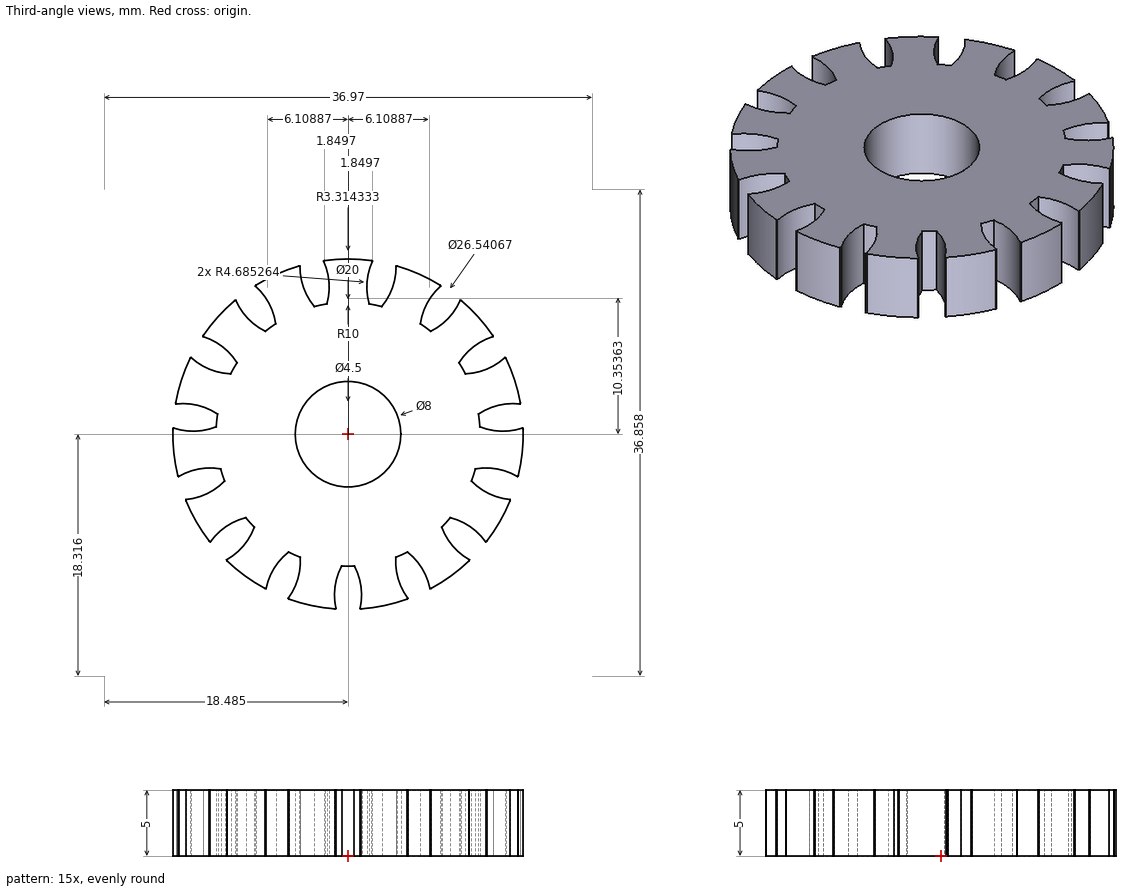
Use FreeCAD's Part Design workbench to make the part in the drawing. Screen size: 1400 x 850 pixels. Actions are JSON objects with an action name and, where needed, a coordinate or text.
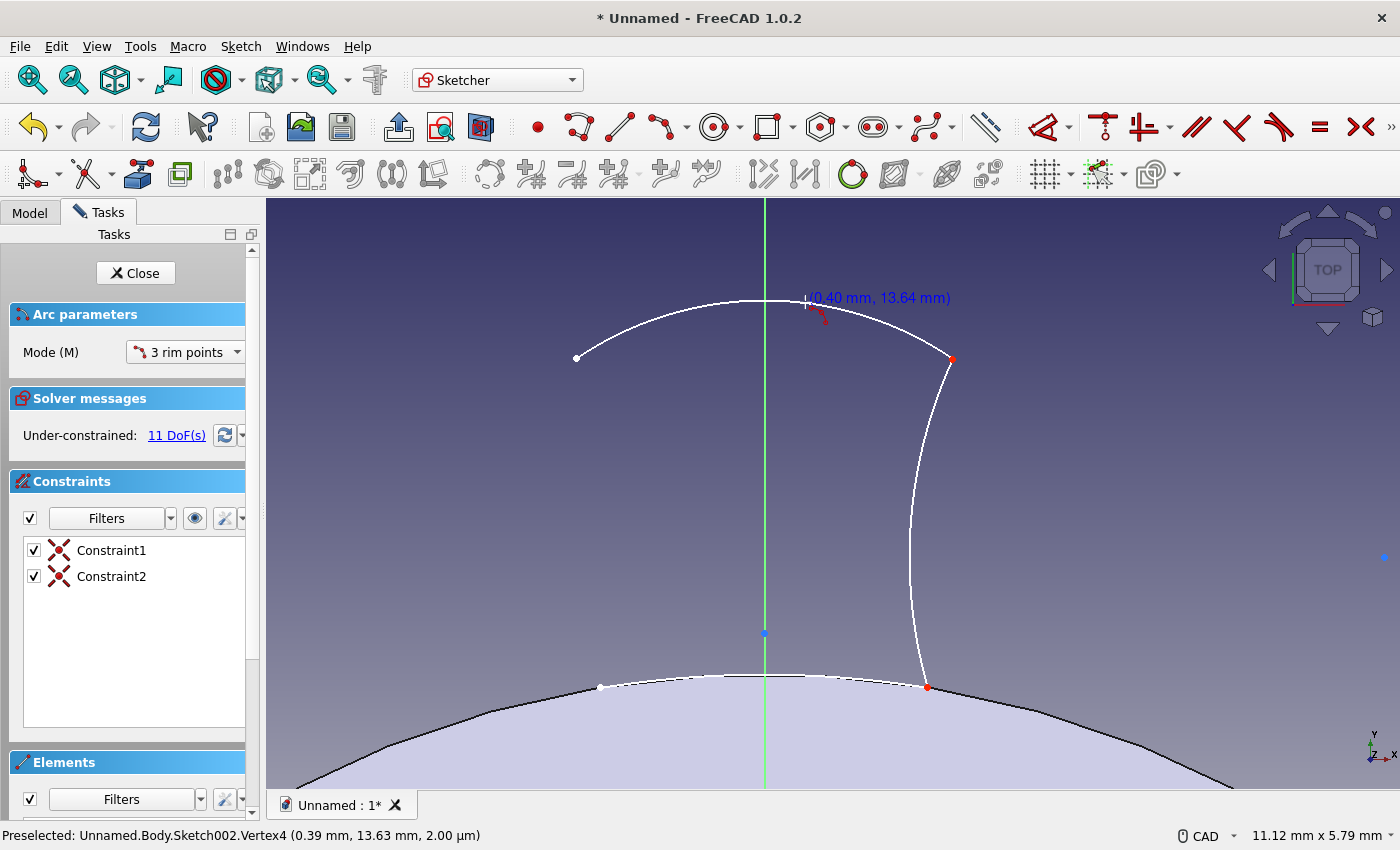
{"action": "left_click", "coordinate": [576, 359]}
{"action": "left_click", "coordinate": [601, 688]}
{"action": "left_click", "coordinate": [618, 520]}
{"action": "key", "text": "Escape"}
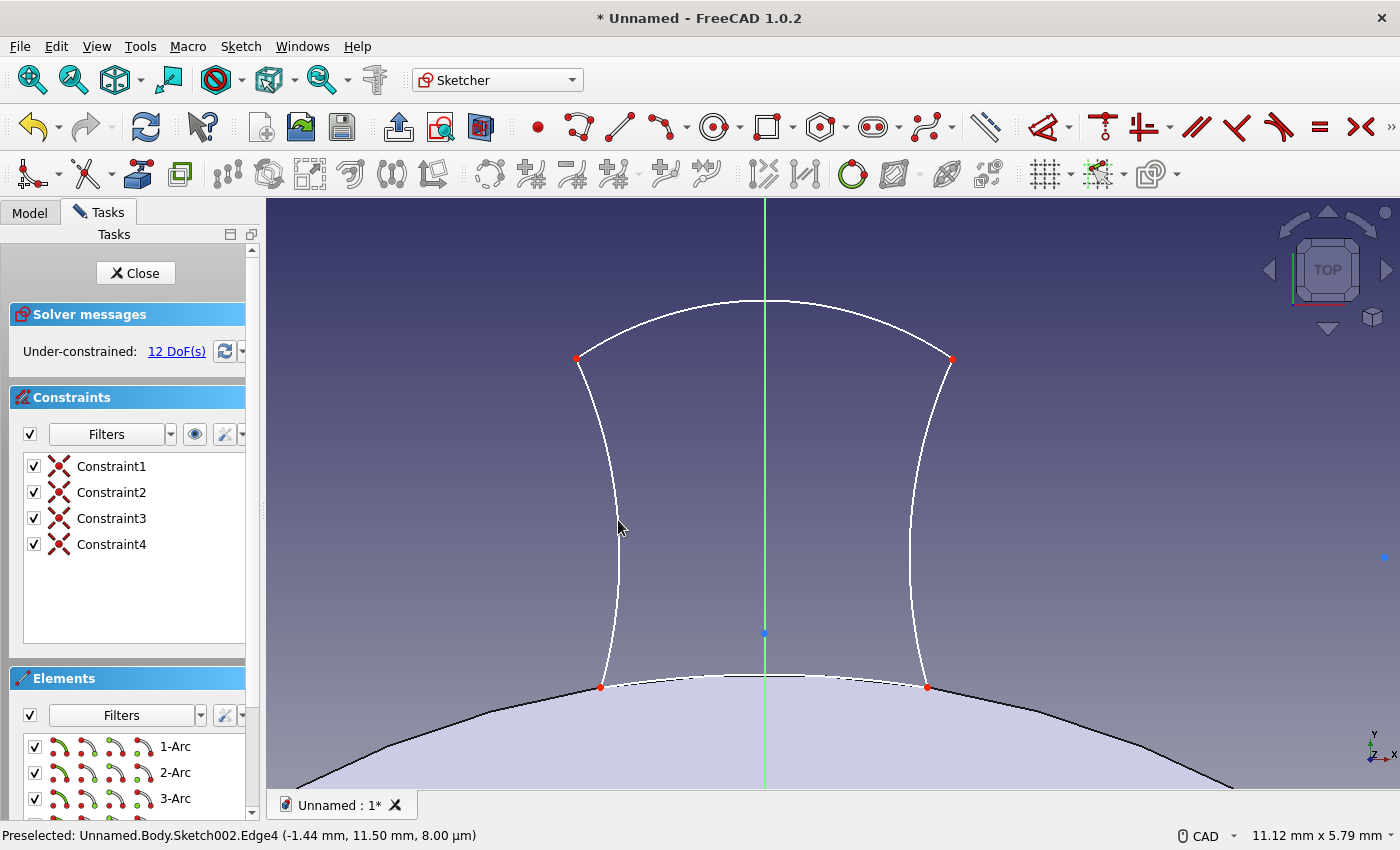
{"action": "scroll", "coordinate": [764, 329], "scroll_direction": "down", "scroll_amount": 7}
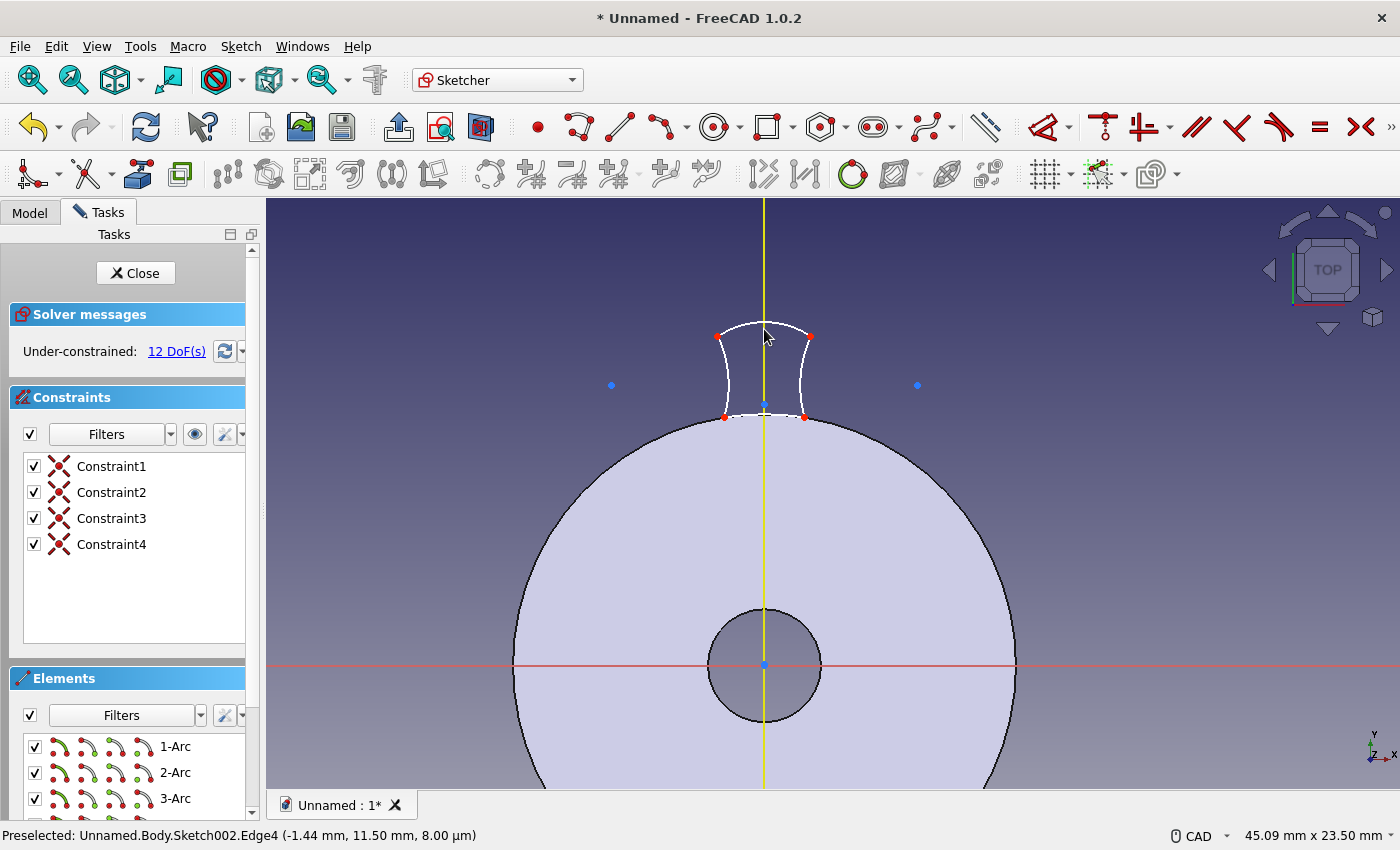
{"action": "left_click_drag", "start_coordinate": [754, 654], "coordinate": [774, 676]}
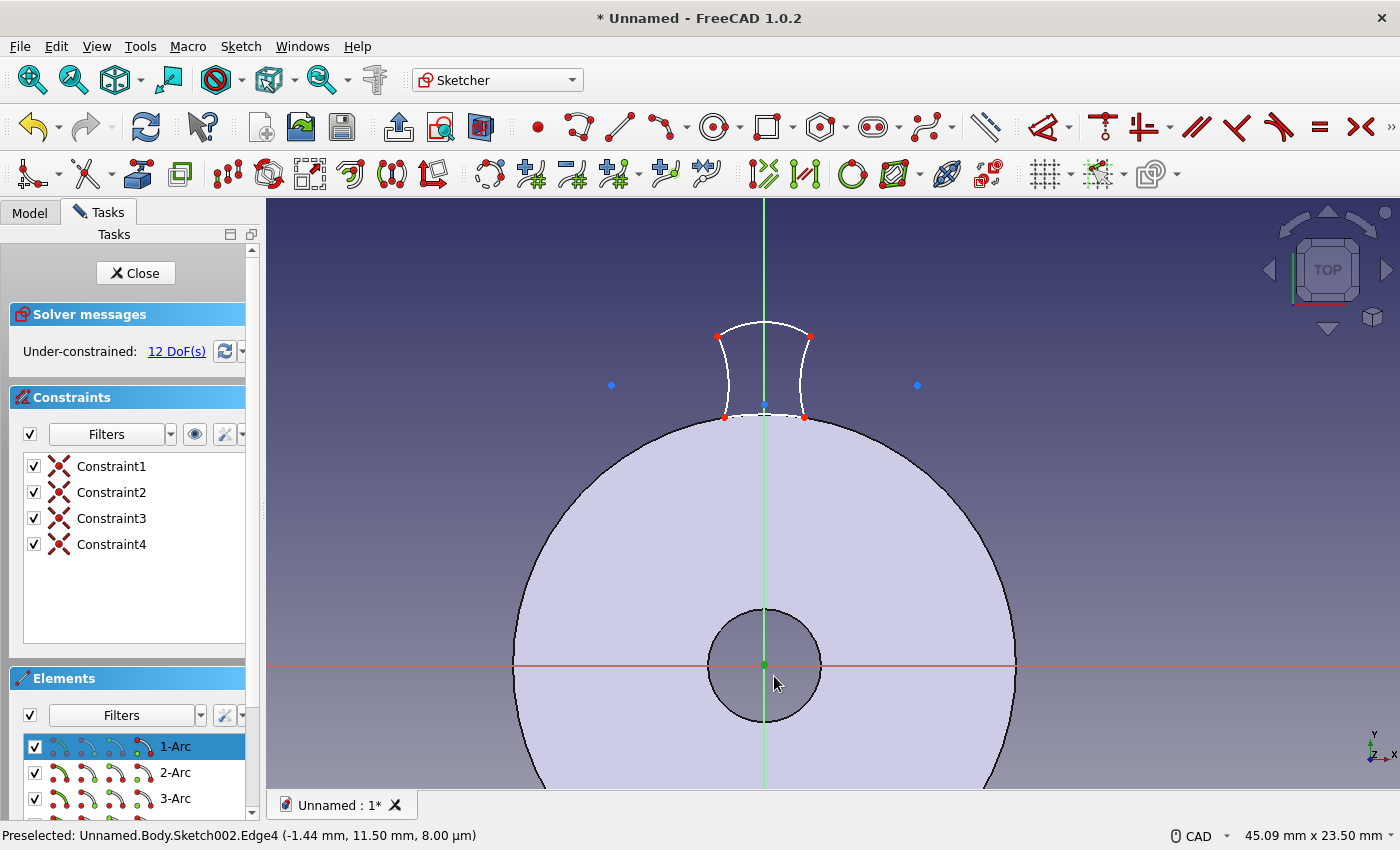
{"action": "key", "text": "c"}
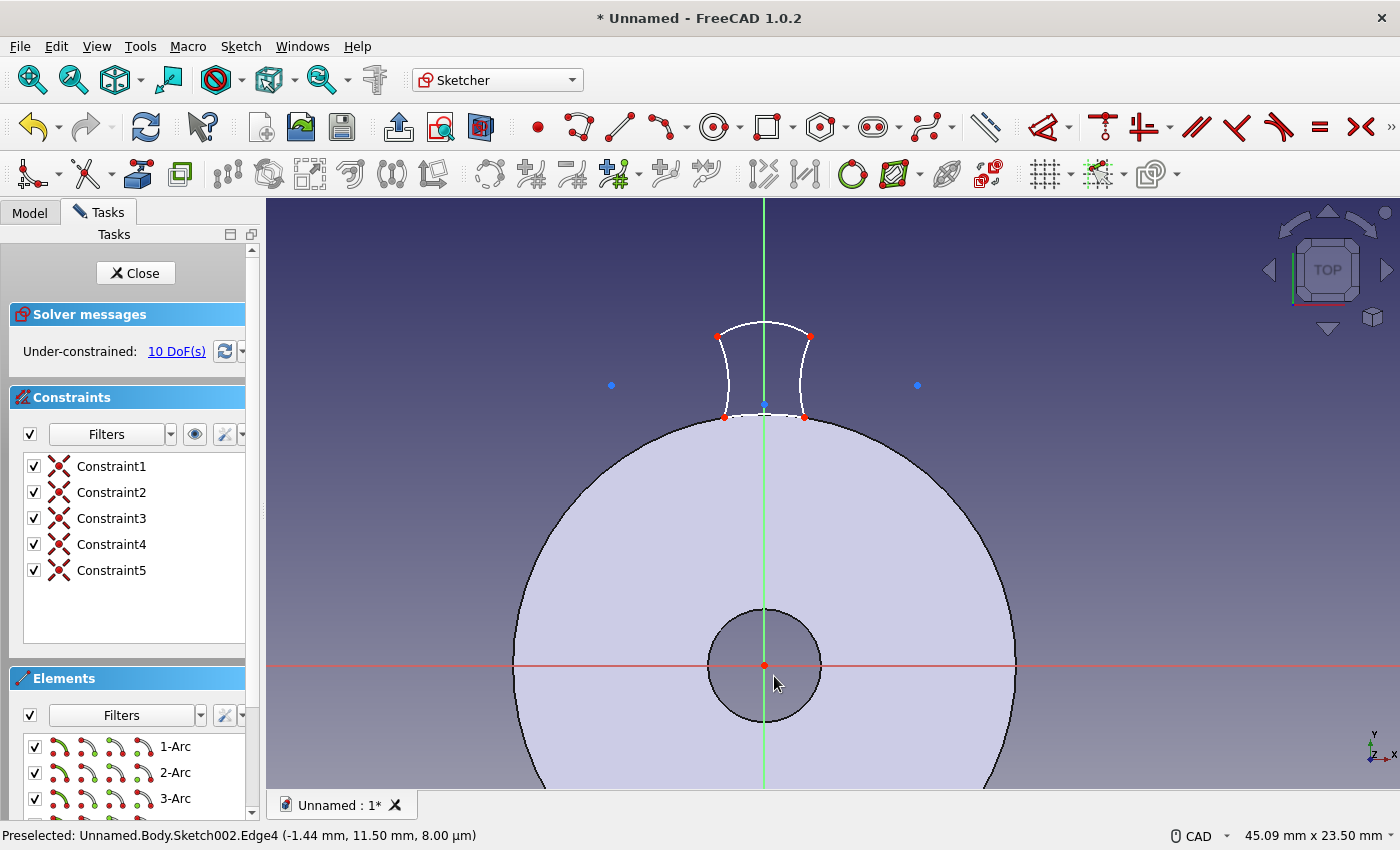
{"action": "left_click", "coordinate": [803, 360]}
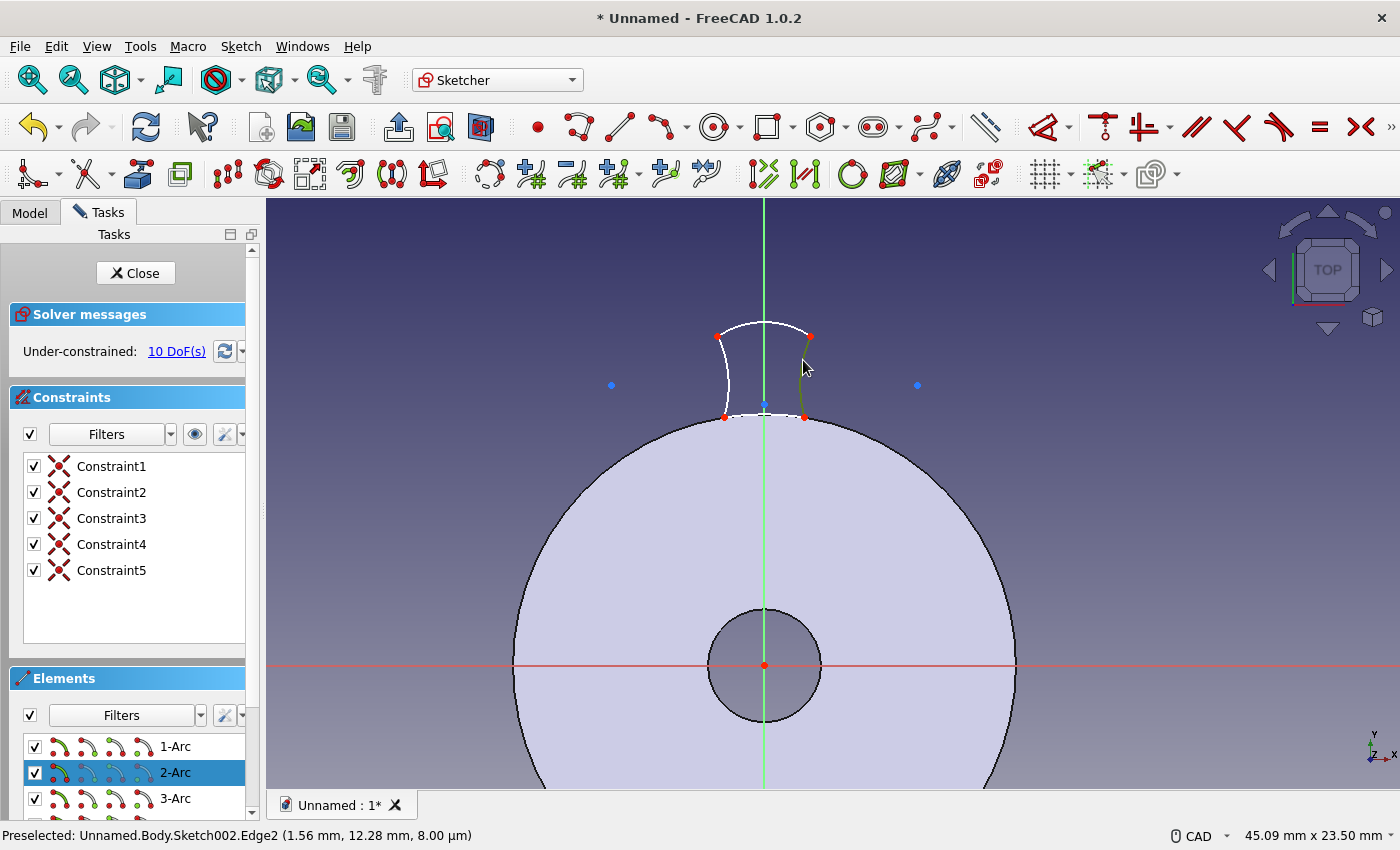
{"action": "left_click", "coordinate": [728, 393]}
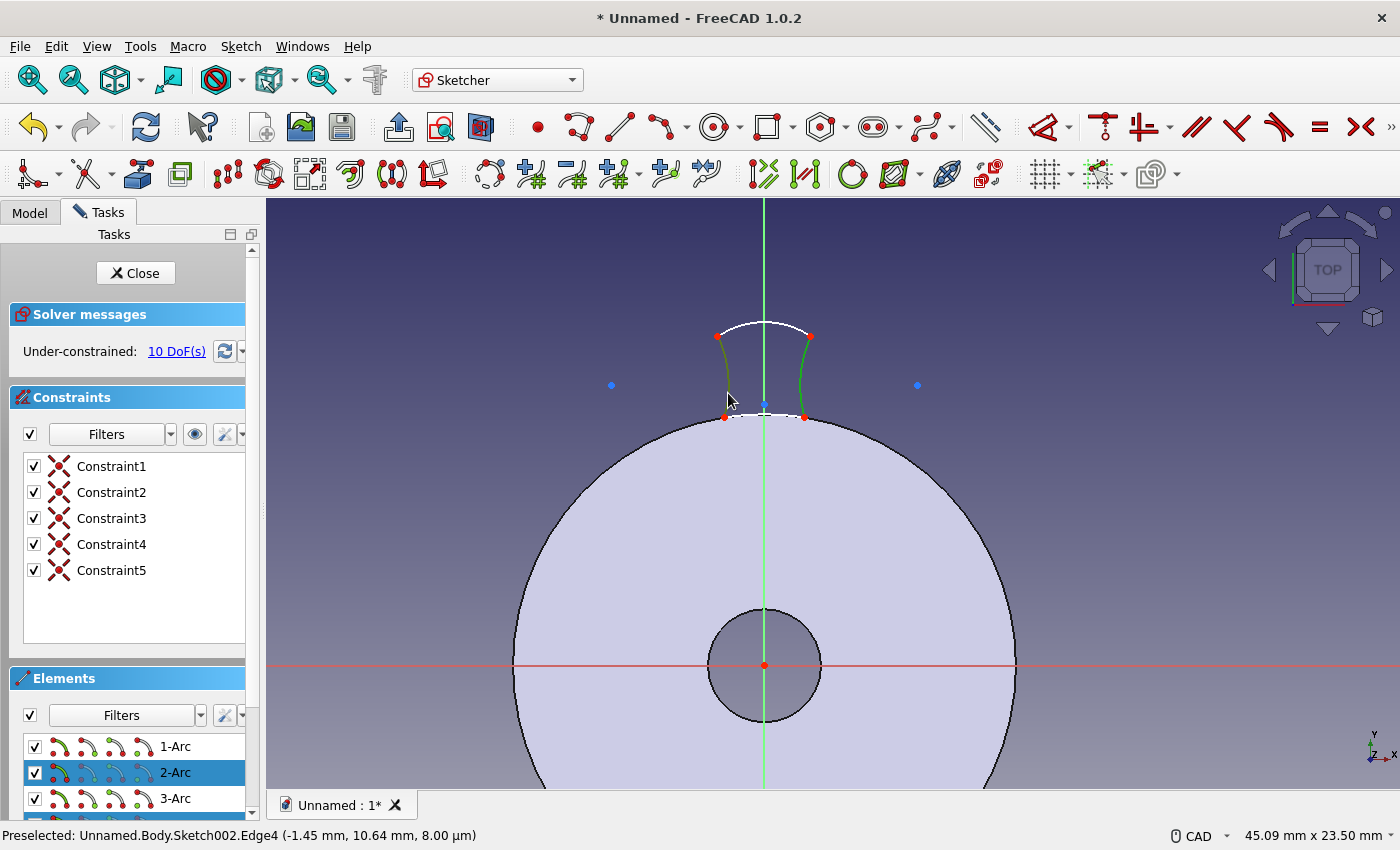
{"action": "left_click", "coordinate": [1320, 128]}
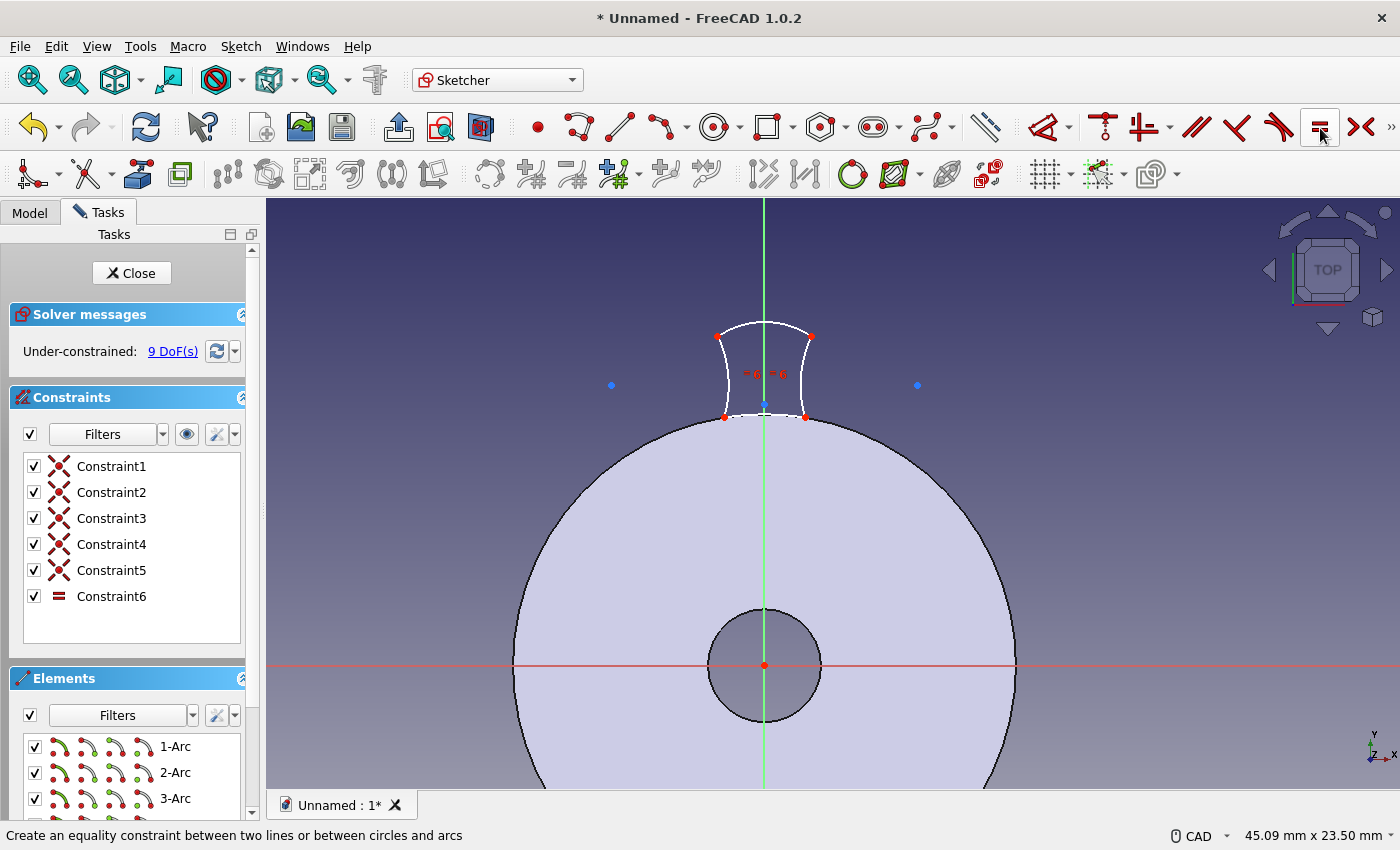
{"action": "left_click", "coordinate": [765, 404]}